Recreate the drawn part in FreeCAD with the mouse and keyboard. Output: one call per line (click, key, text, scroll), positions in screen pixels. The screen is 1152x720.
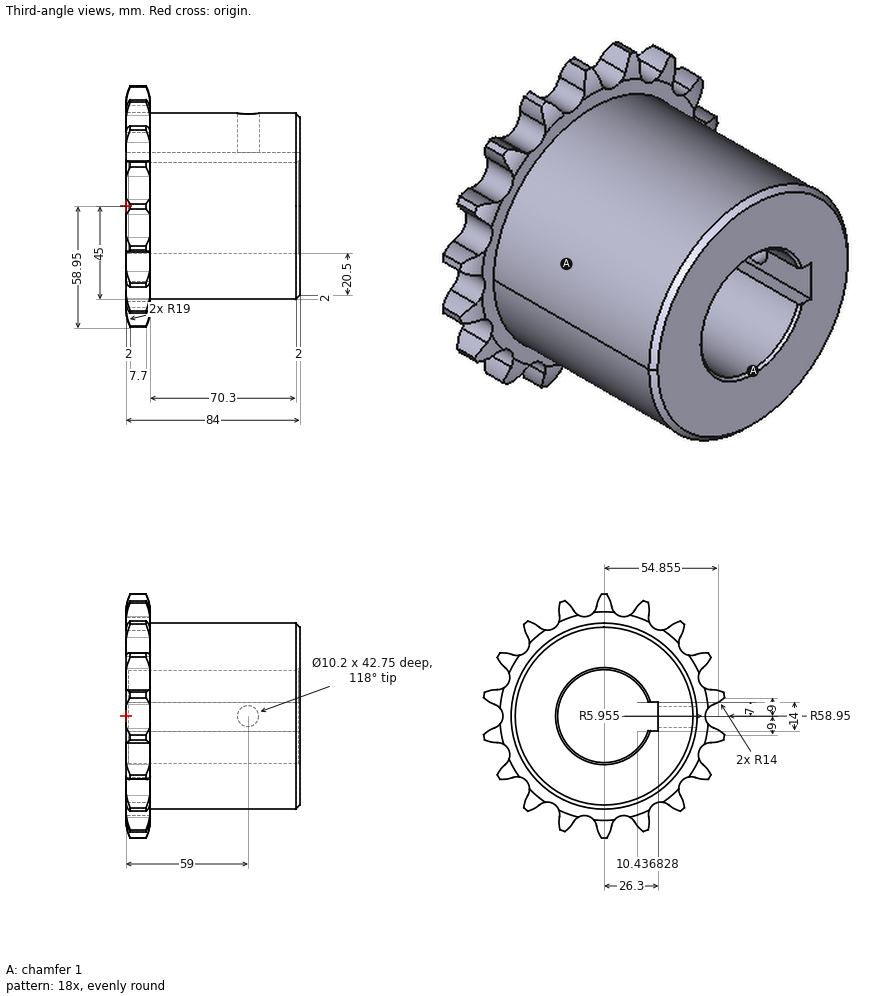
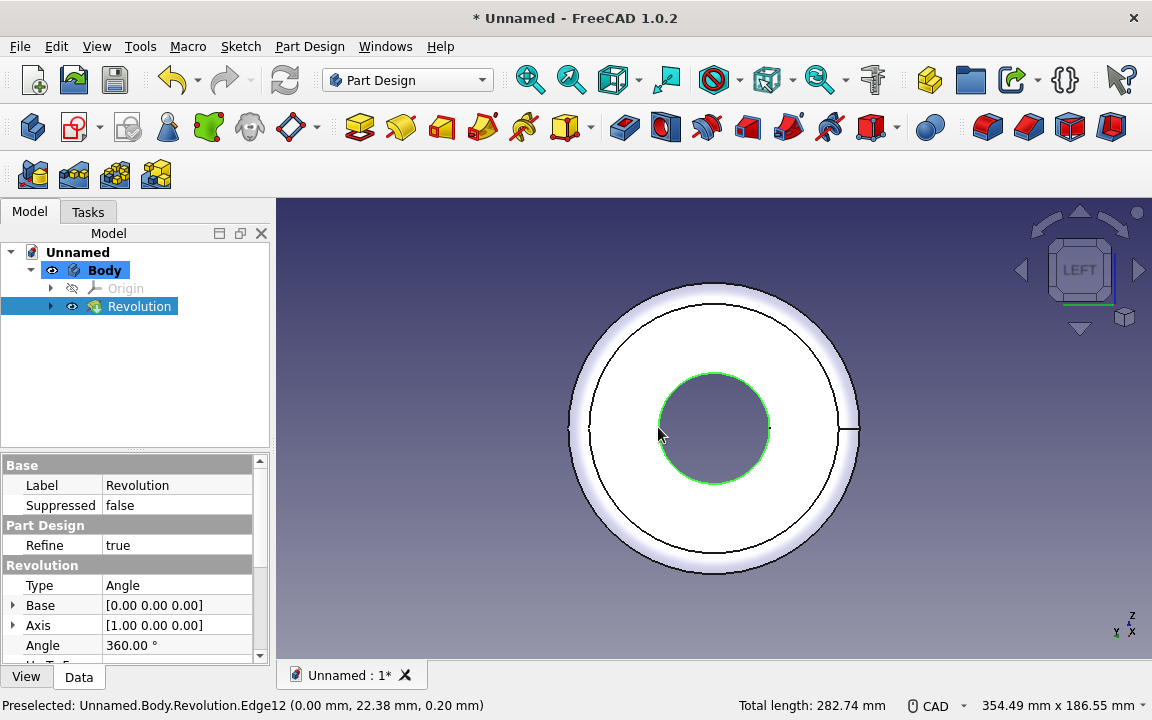
click(1029, 128)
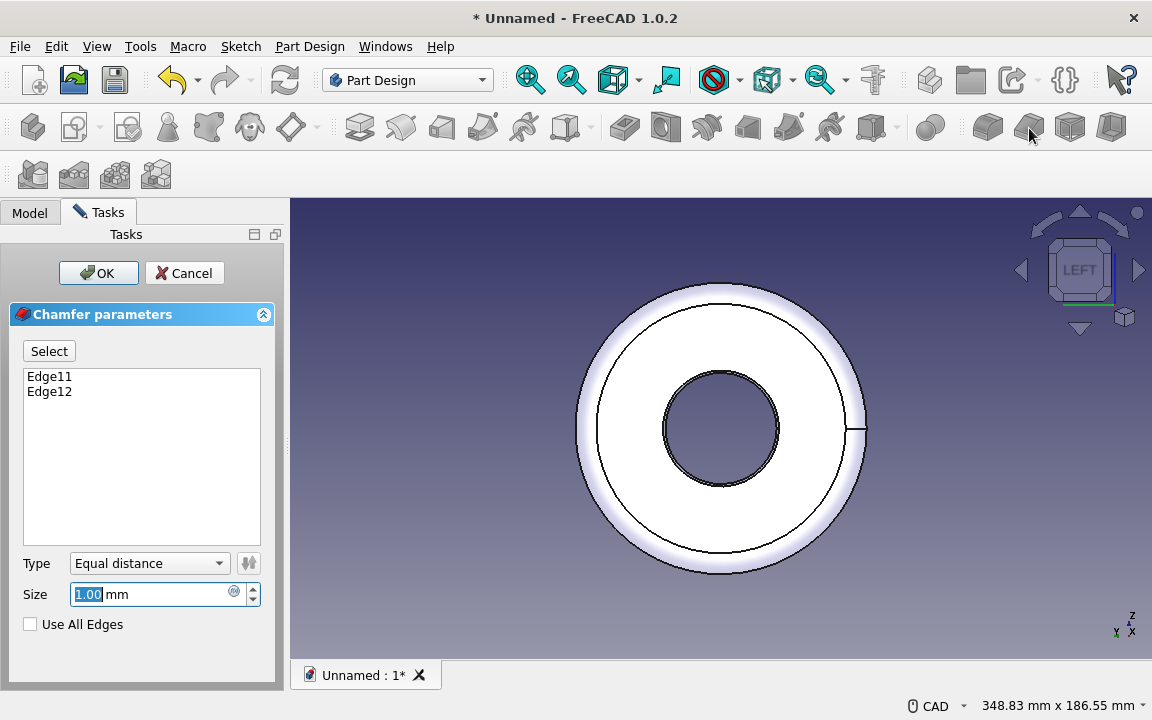
text(1)
key(Tab)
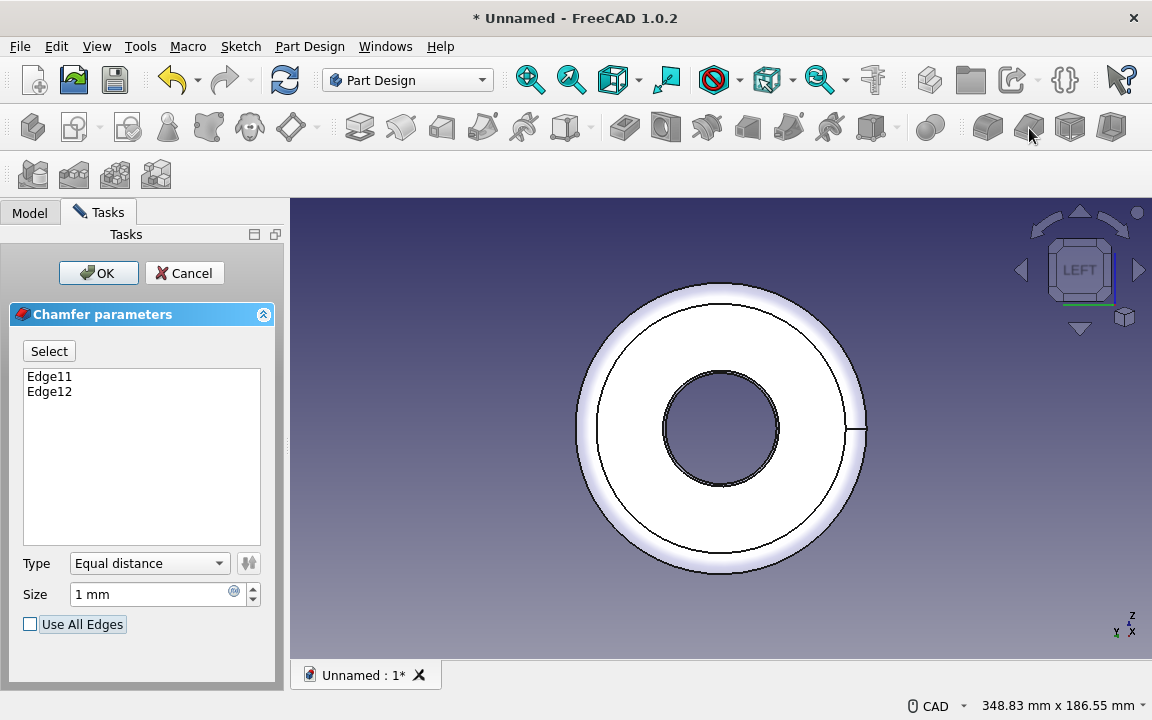
click(99, 273)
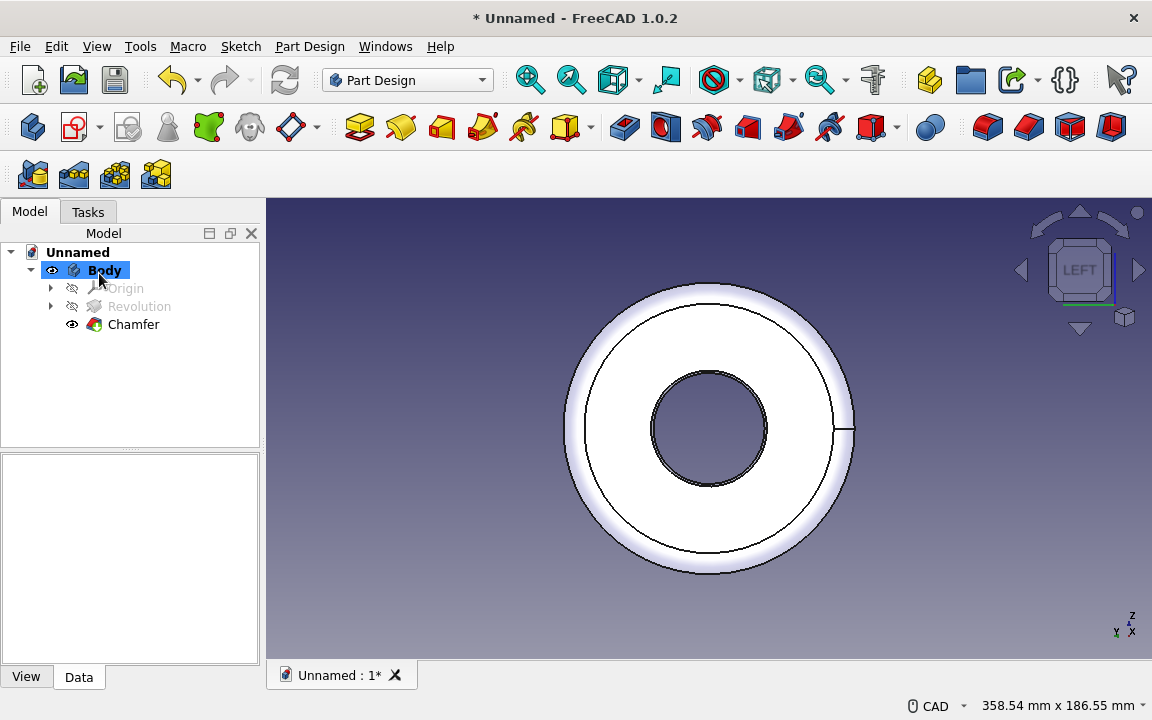
key(0)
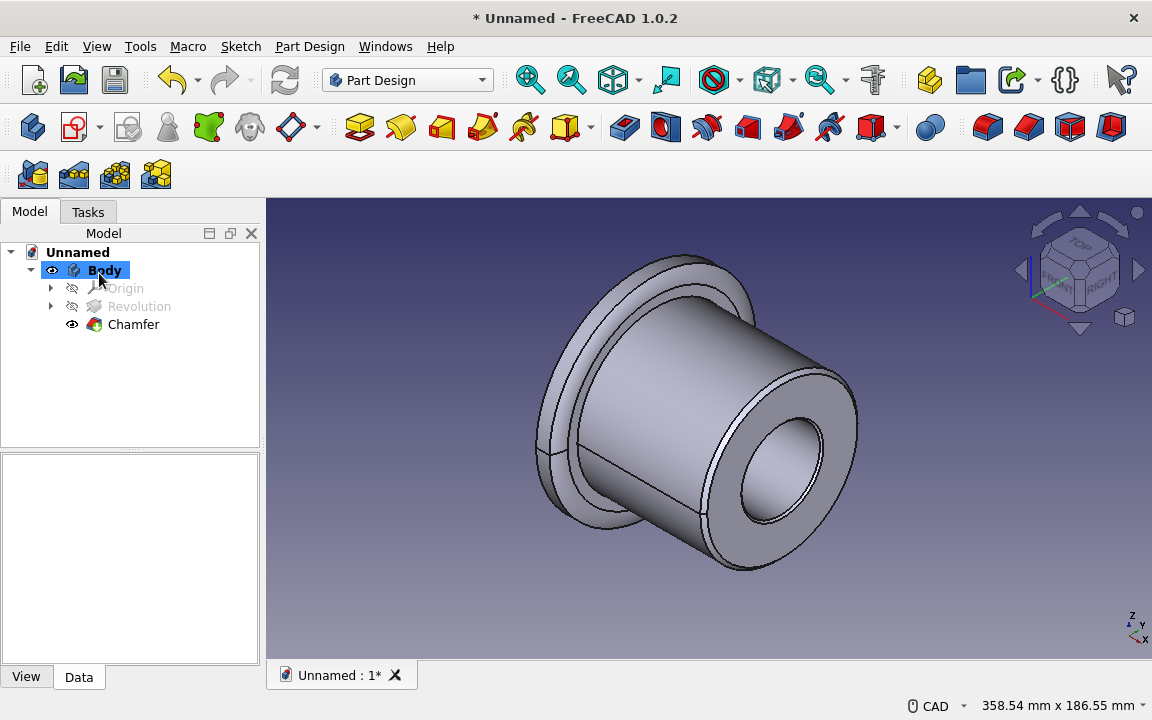
click(825, 495)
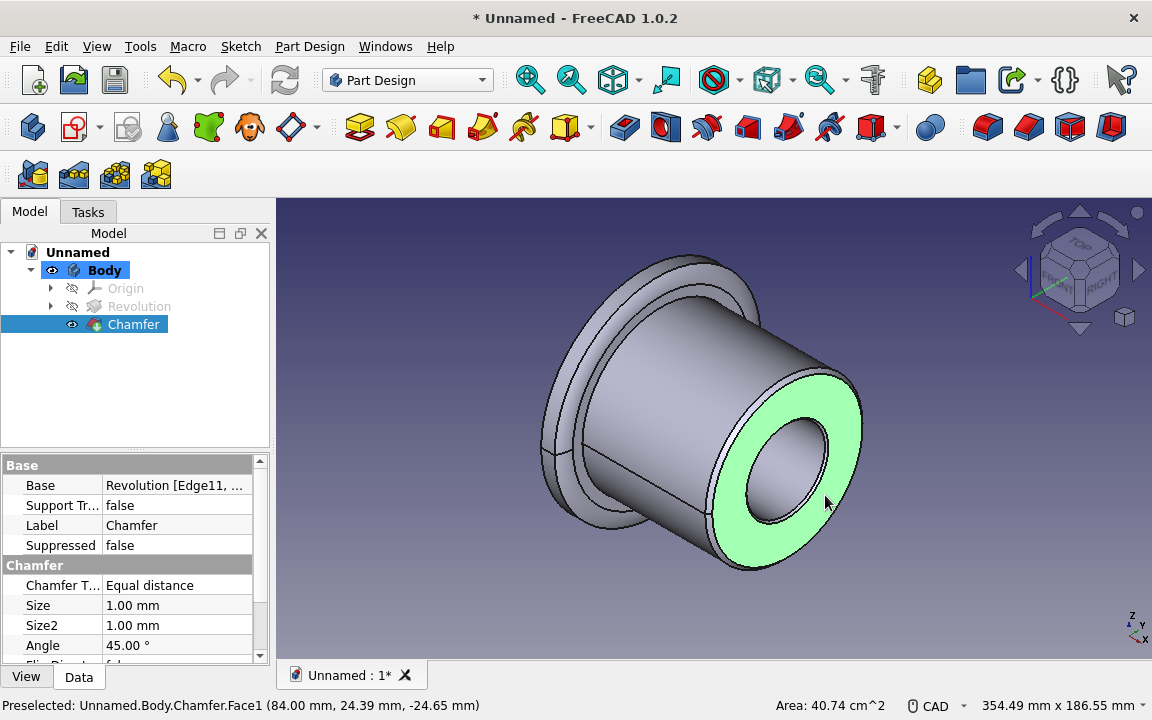
click(74, 128)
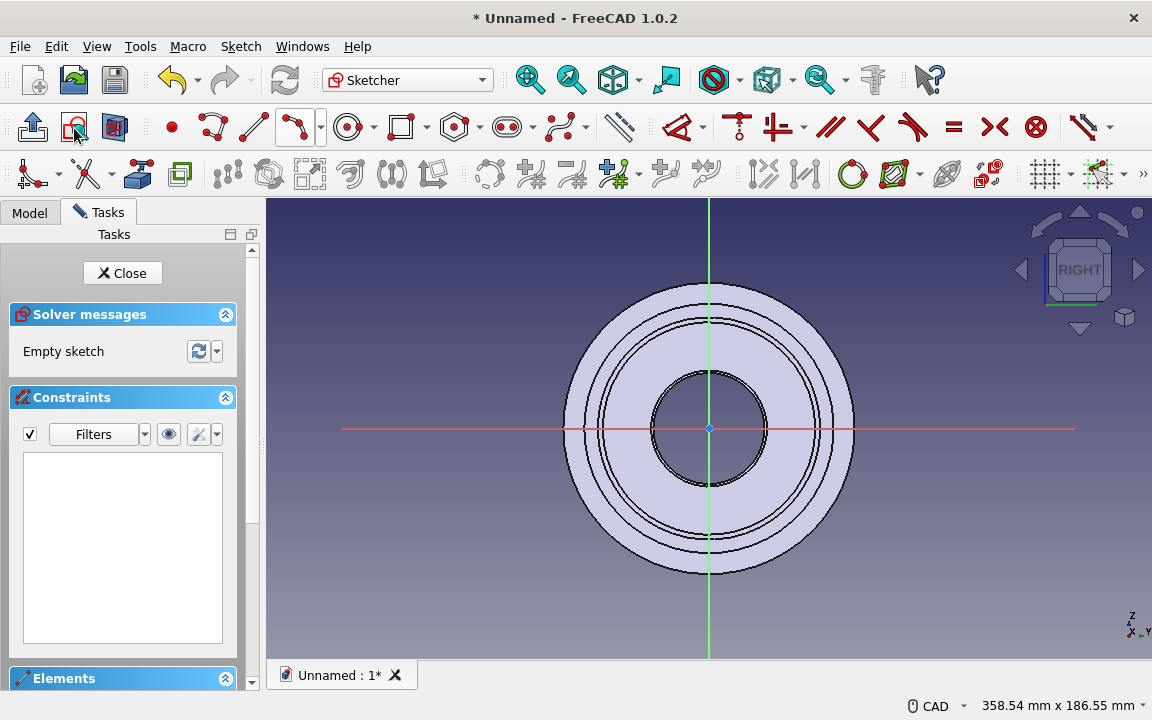
scroll(757, 428, up, 10)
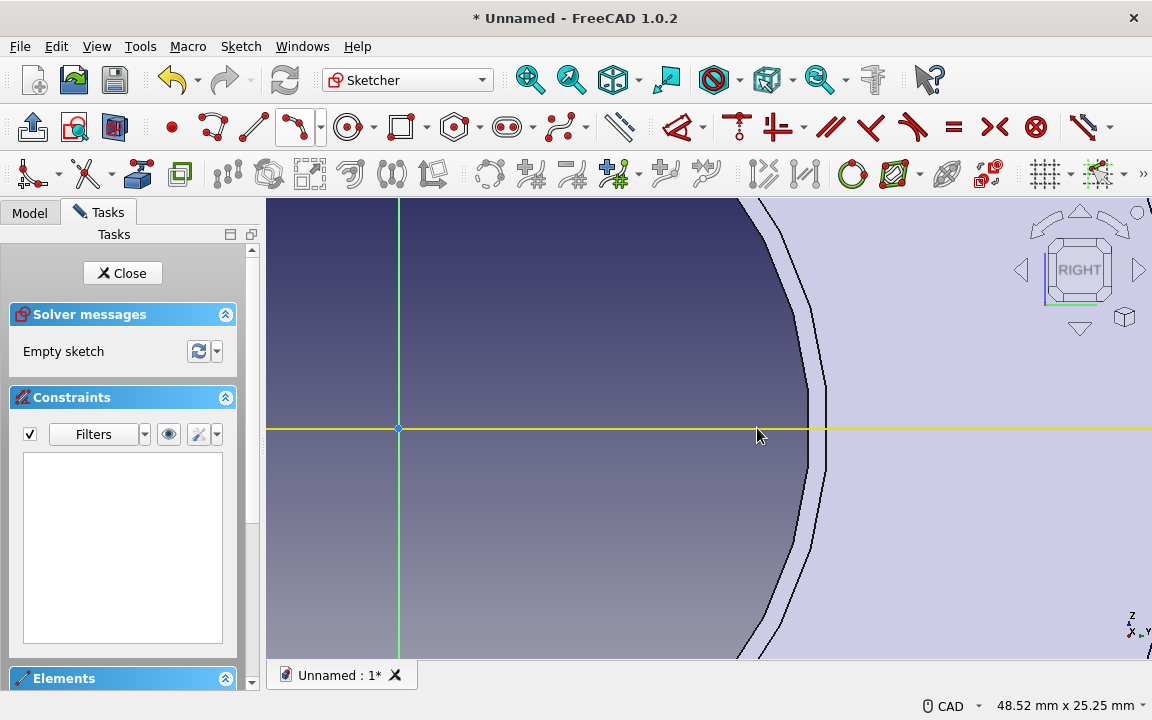
click(400, 128)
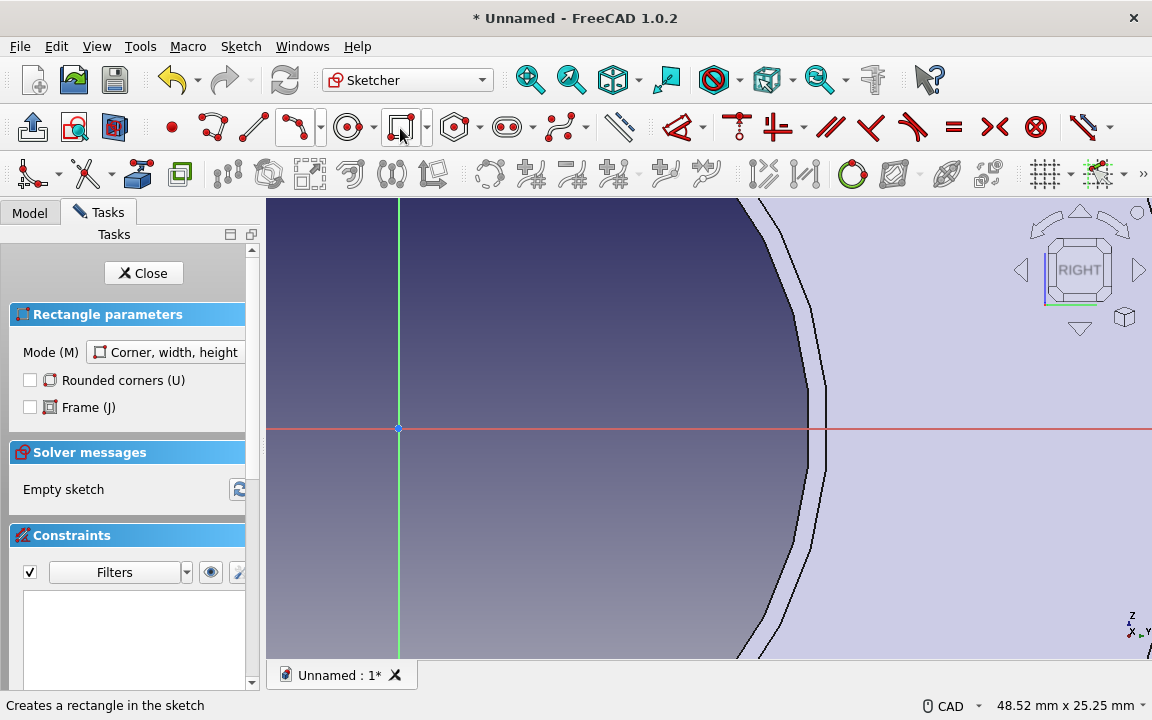
click(688, 301)
click(879, 556)
key(Escape)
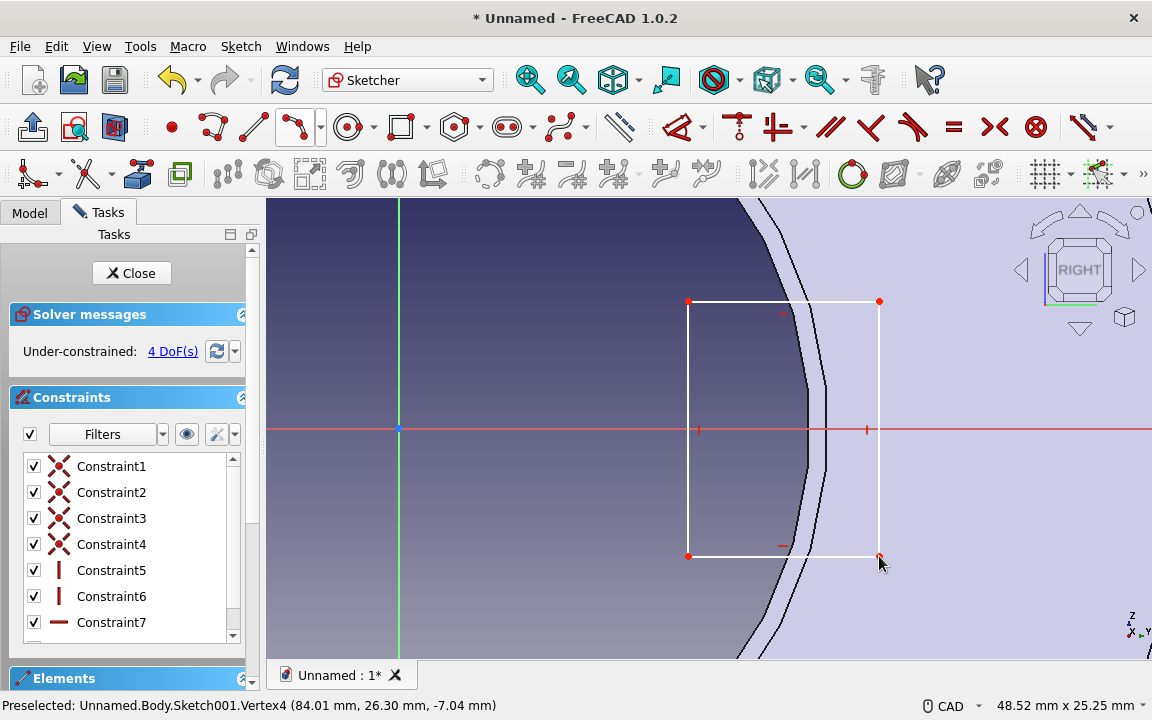
click(676, 128)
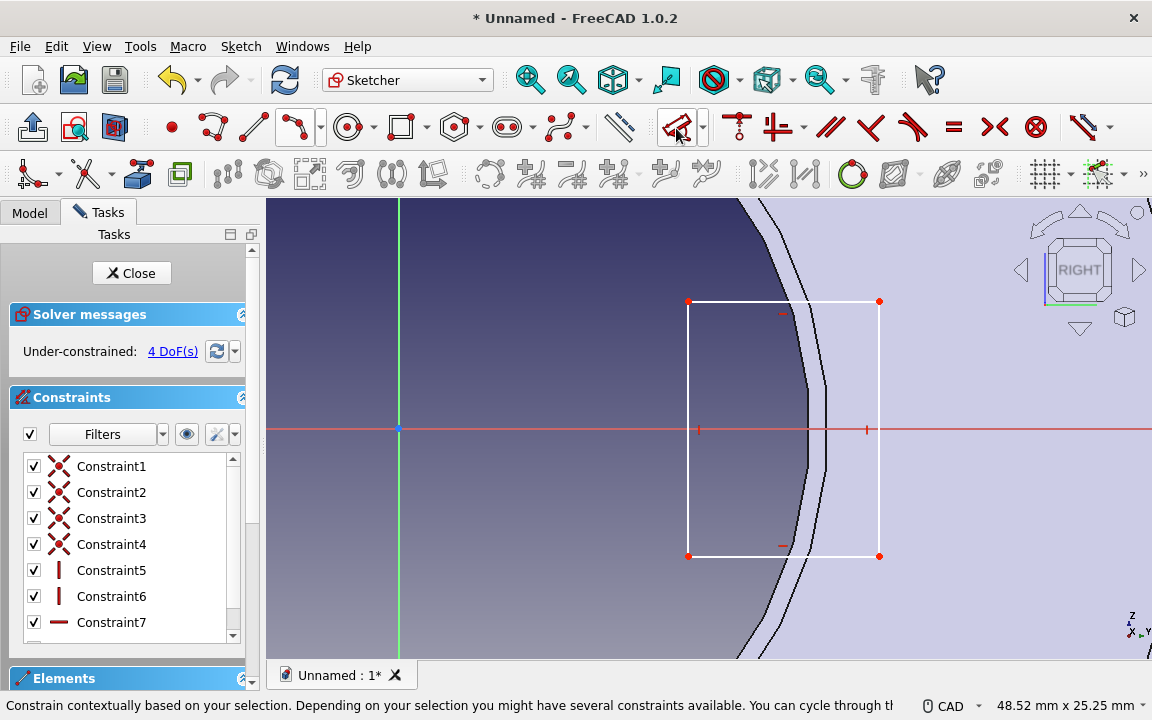
click(688, 379)
click(722, 371)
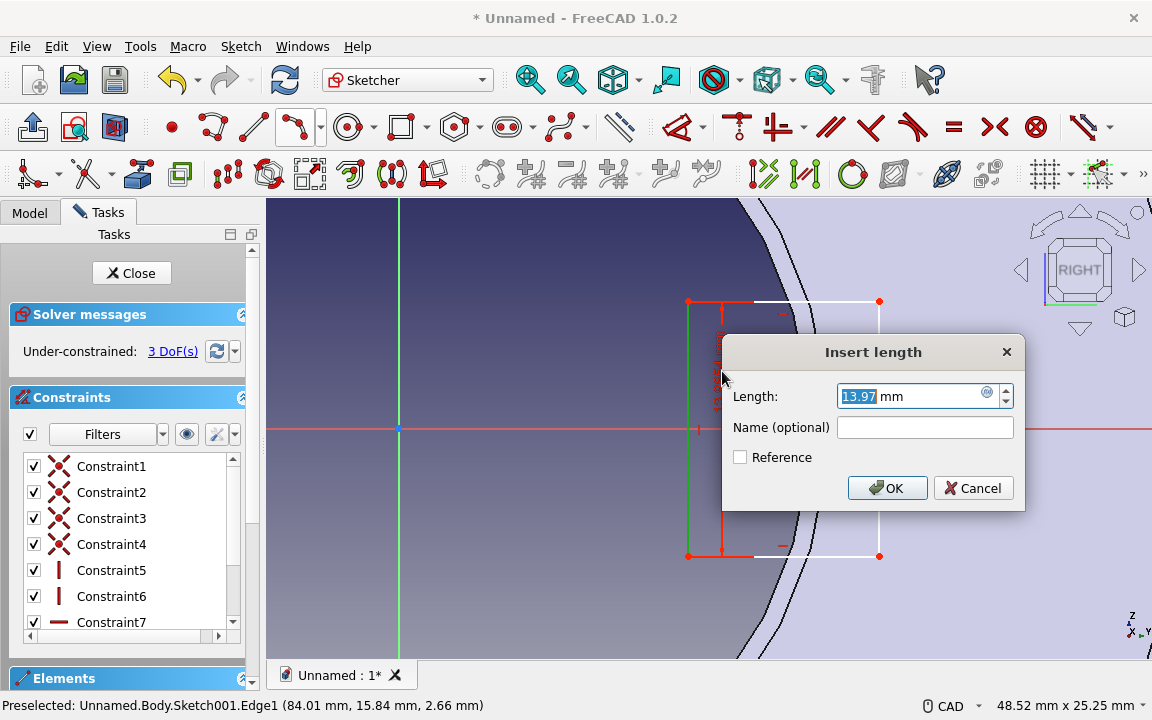
text(14)
key(Return)